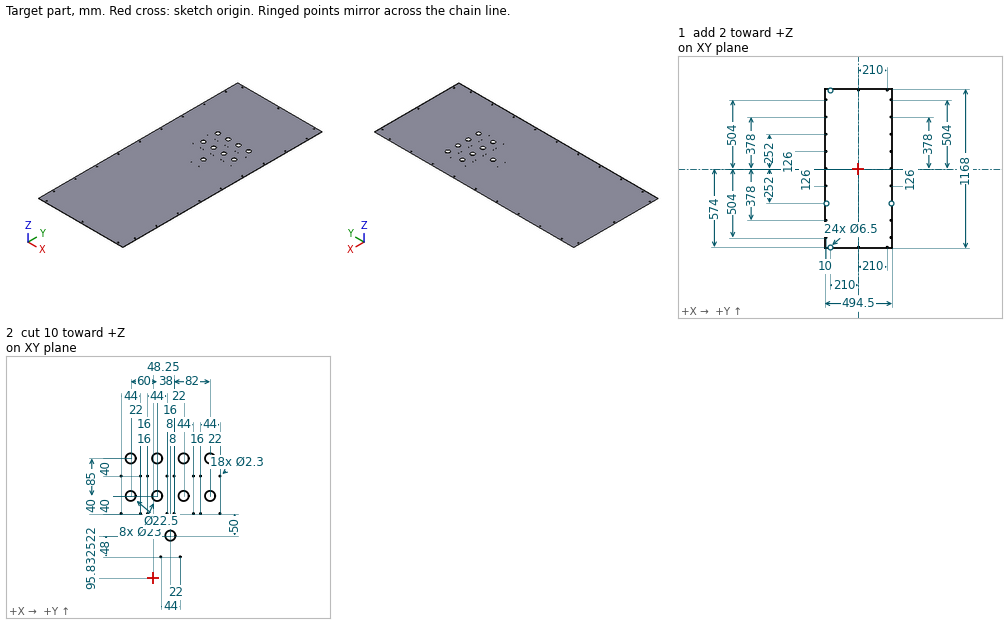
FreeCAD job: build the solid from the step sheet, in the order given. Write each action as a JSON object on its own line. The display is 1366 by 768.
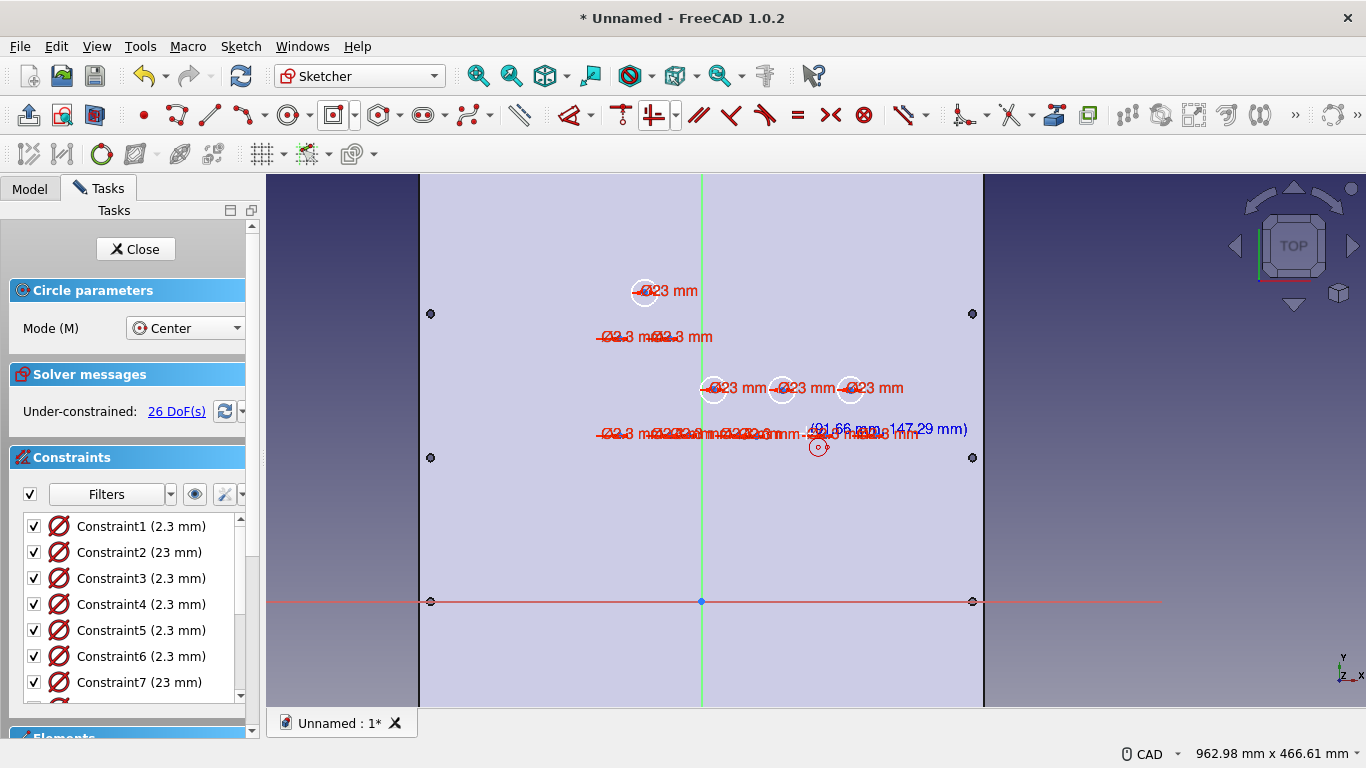
{"action": "left_click", "coordinate": [807, 435]}
{"action": "mouse_move", "coordinate": [808, 434]}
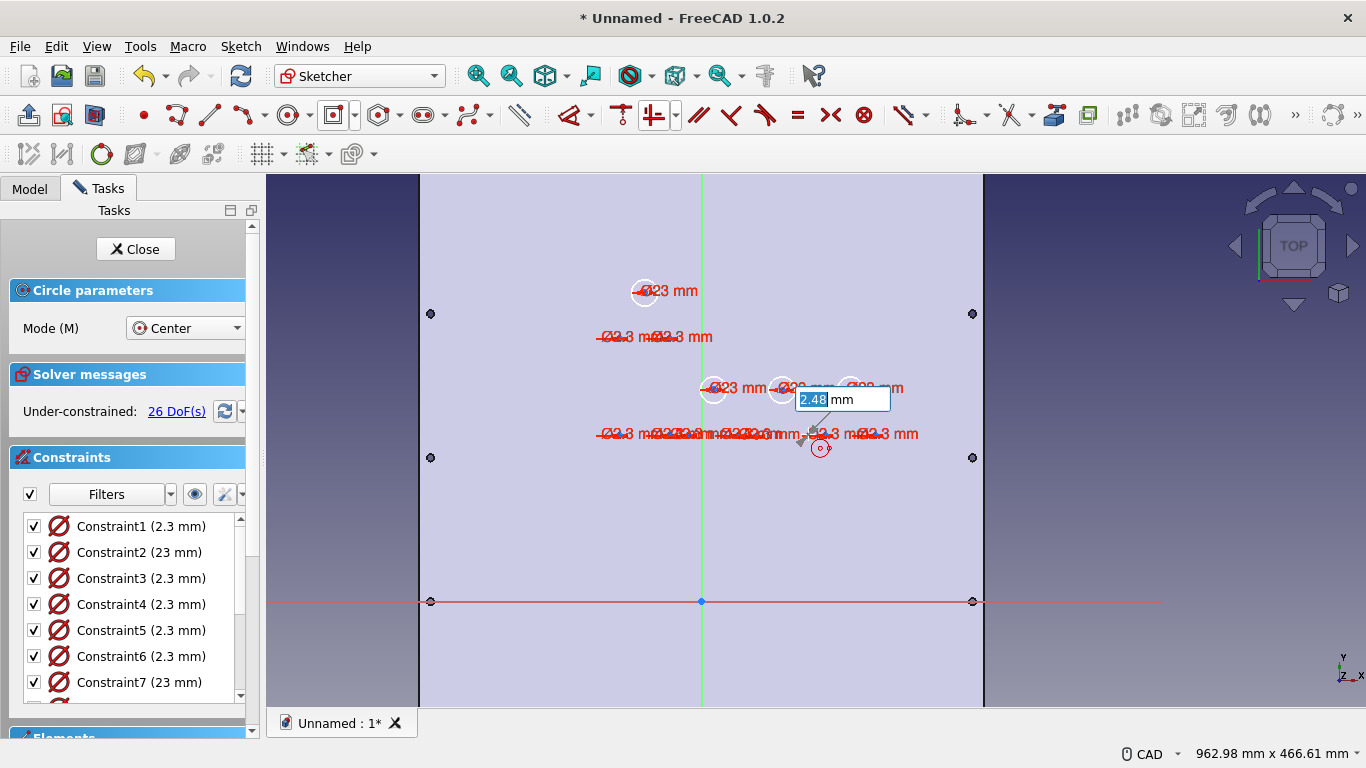
{"action": "type", "text": "2.3"}
{"action": "key", "text": "Return"}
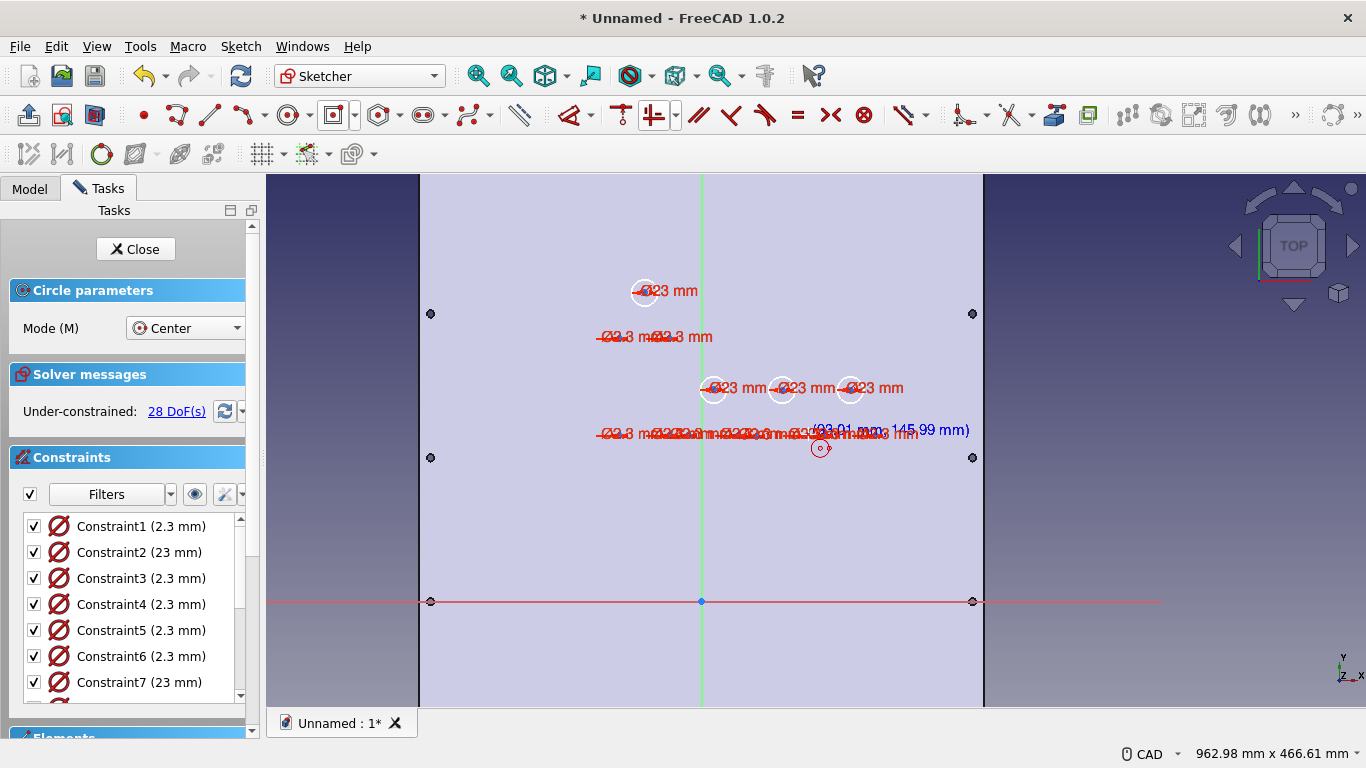
{"action": "scroll", "coordinate": [876, 338], "scroll_direction": "up", "scroll_amount": 15}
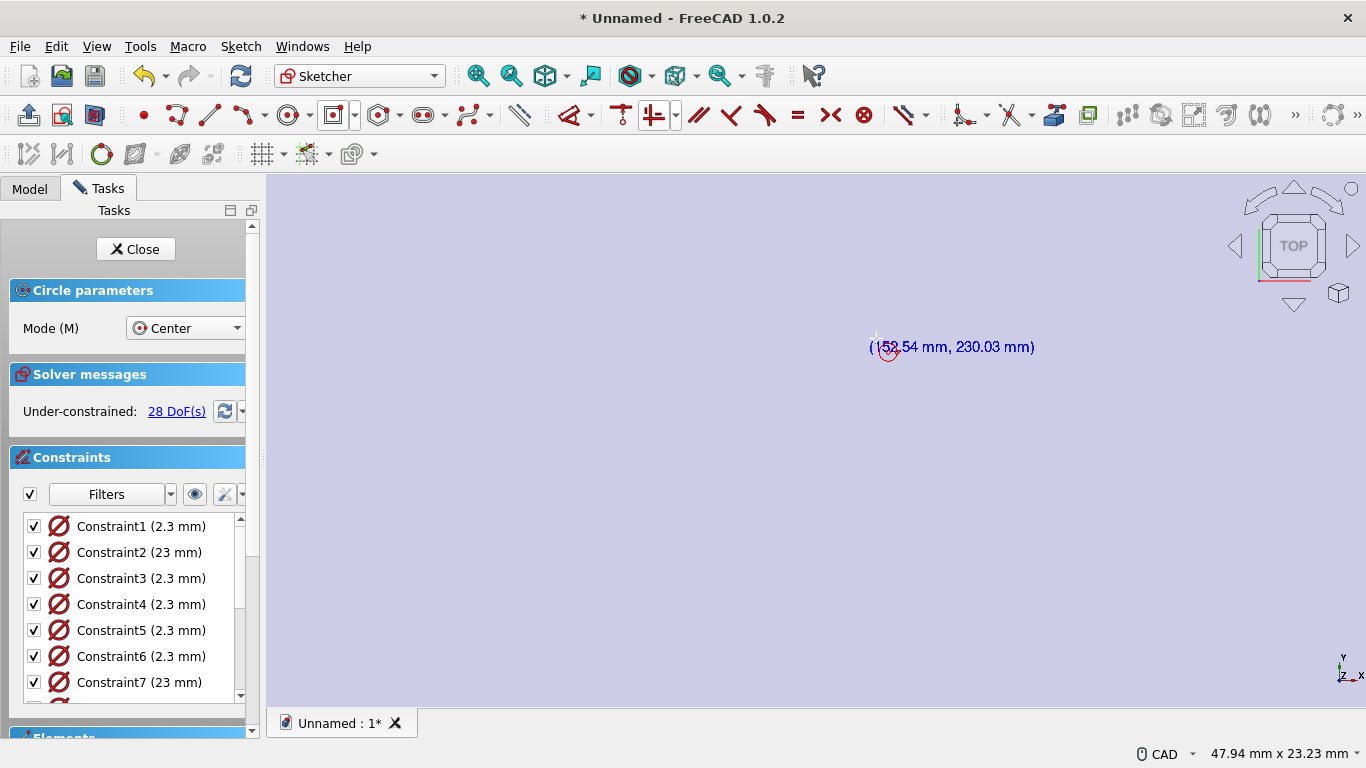
{"action": "scroll", "coordinate": [876, 338], "scroll_direction": "down", "scroll_amount": 15}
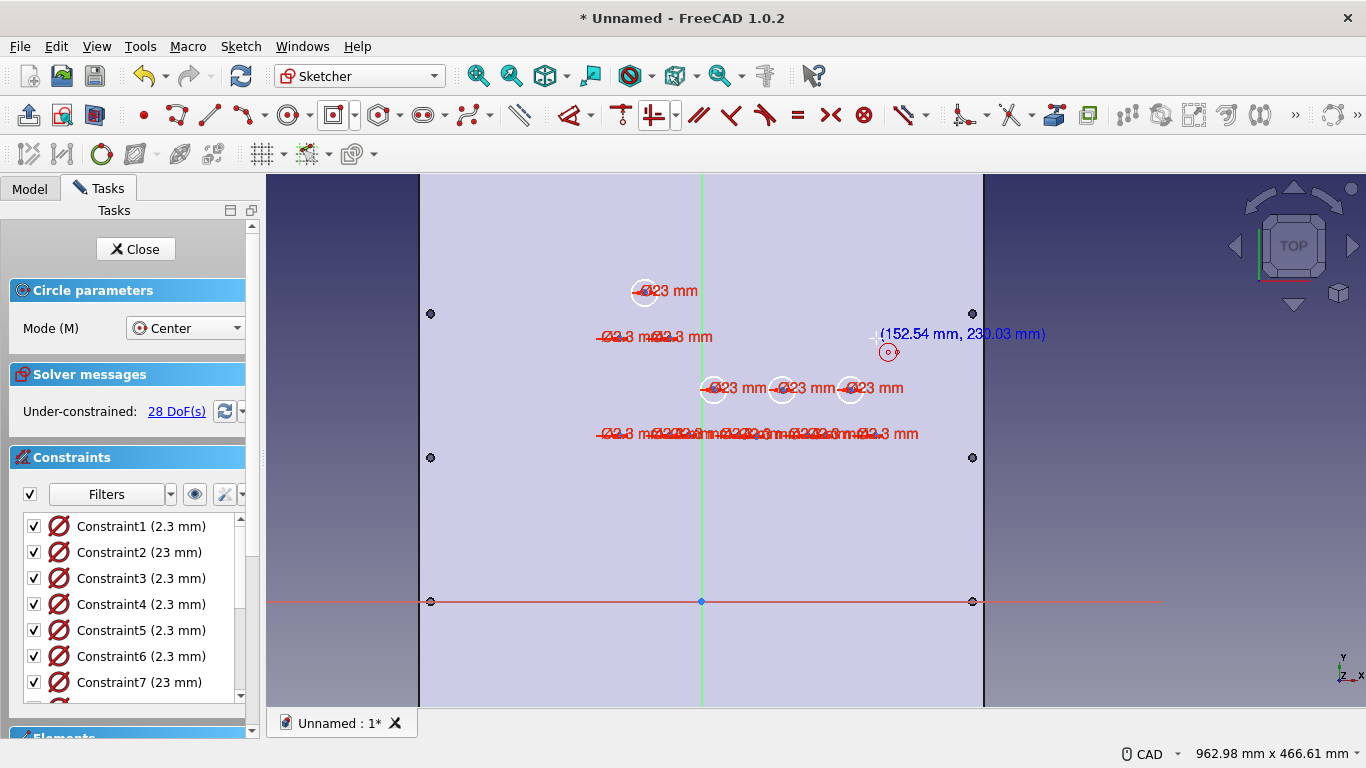
{"action": "left_click", "coordinate": [876, 338]}
{"action": "mouse_move", "coordinate": [877, 337]}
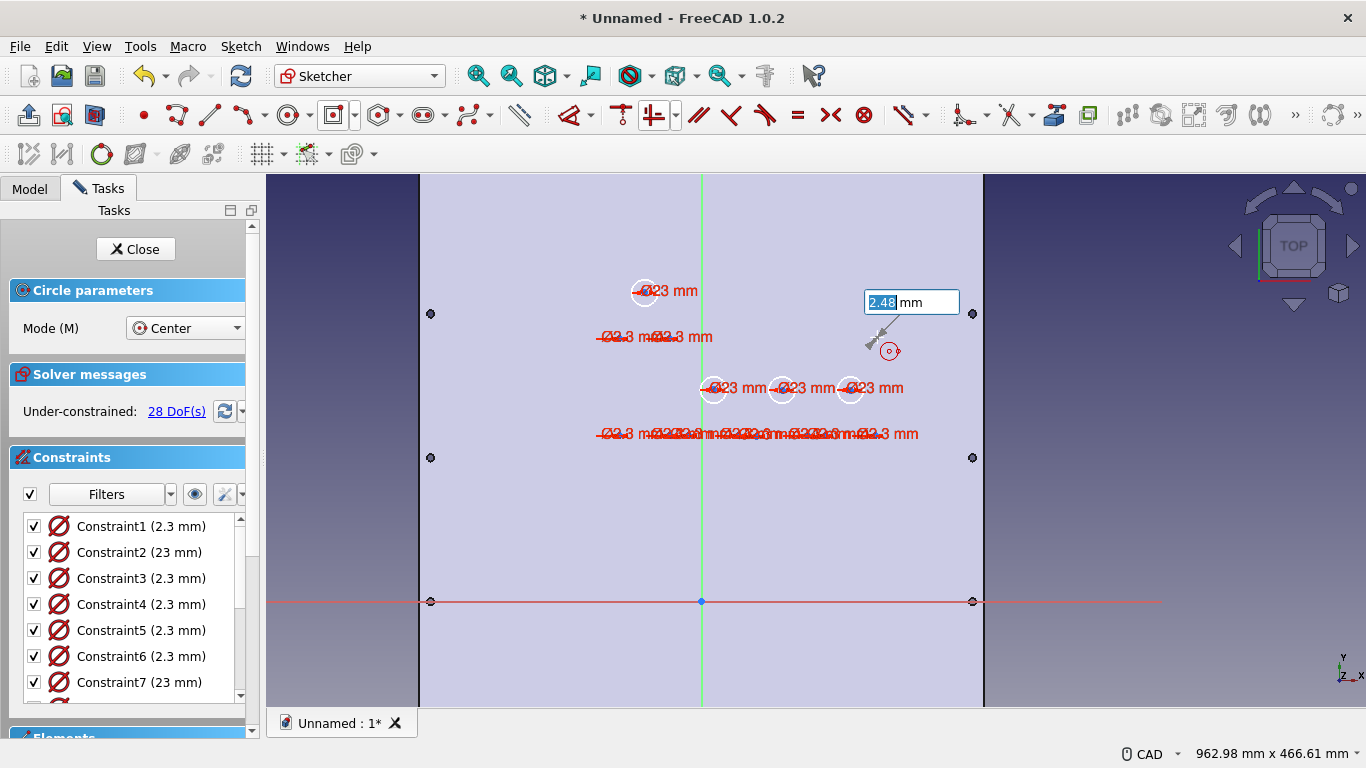
{"action": "type", "text": "2.3"}
{"action": "key", "text": "Return"}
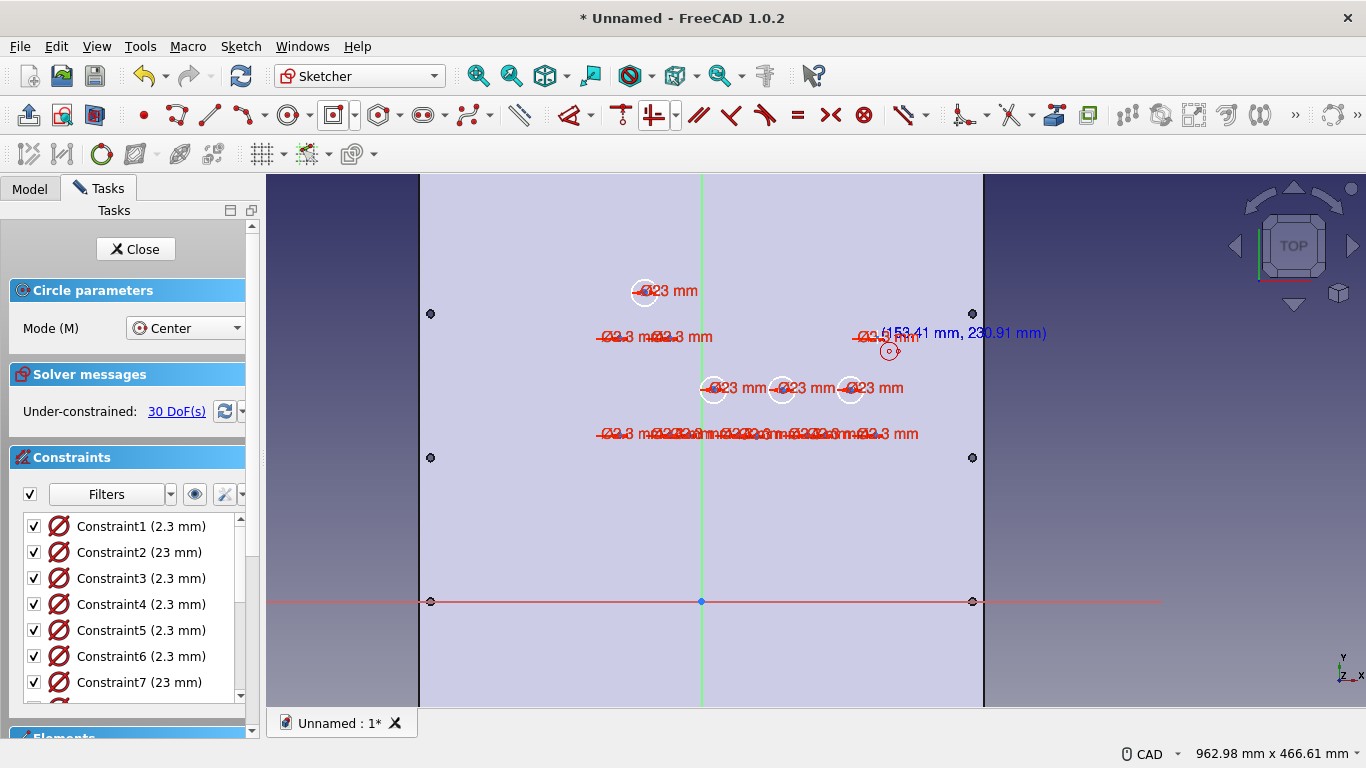
{"action": "scroll", "coordinate": [825, 338], "scroll_direction": "up", "scroll_amount": 15}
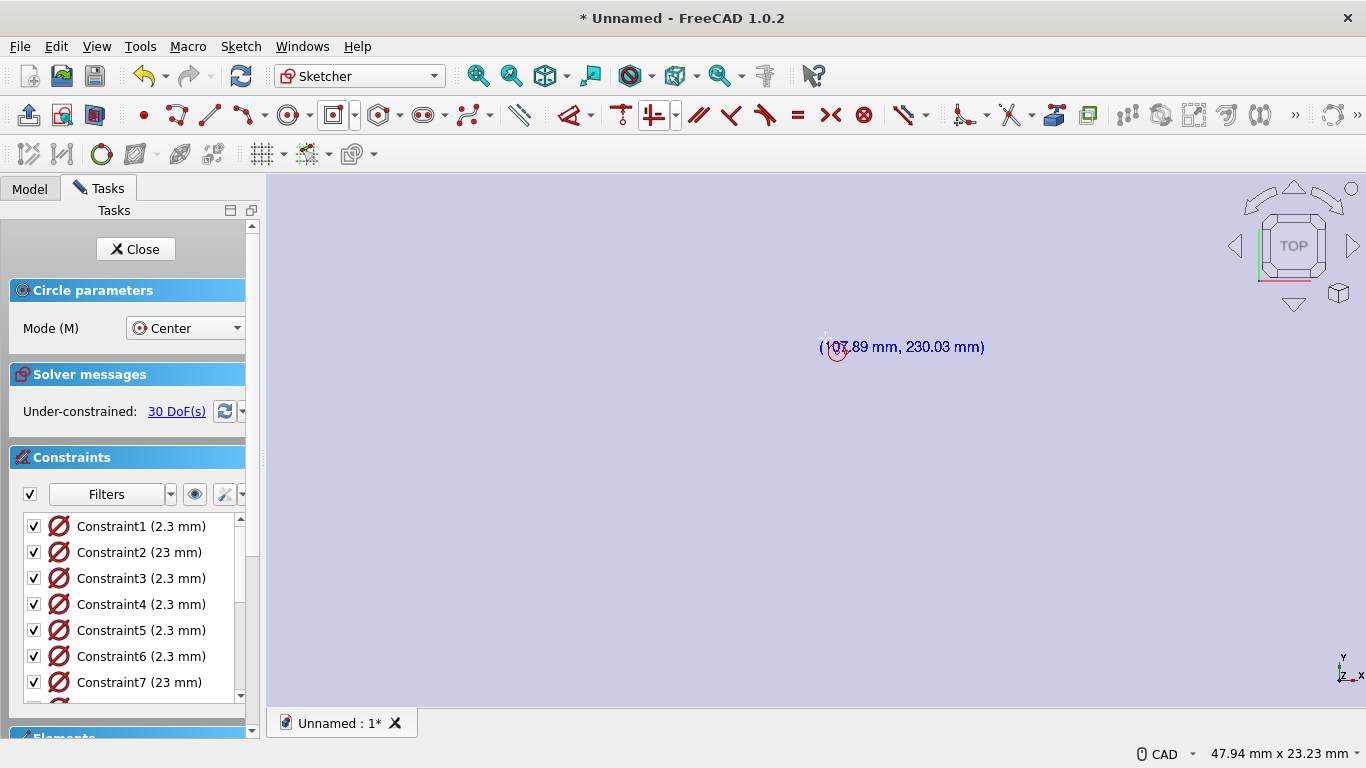
{"action": "scroll", "coordinate": [825, 338], "scroll_direction": "down", "scroll_amount": 15}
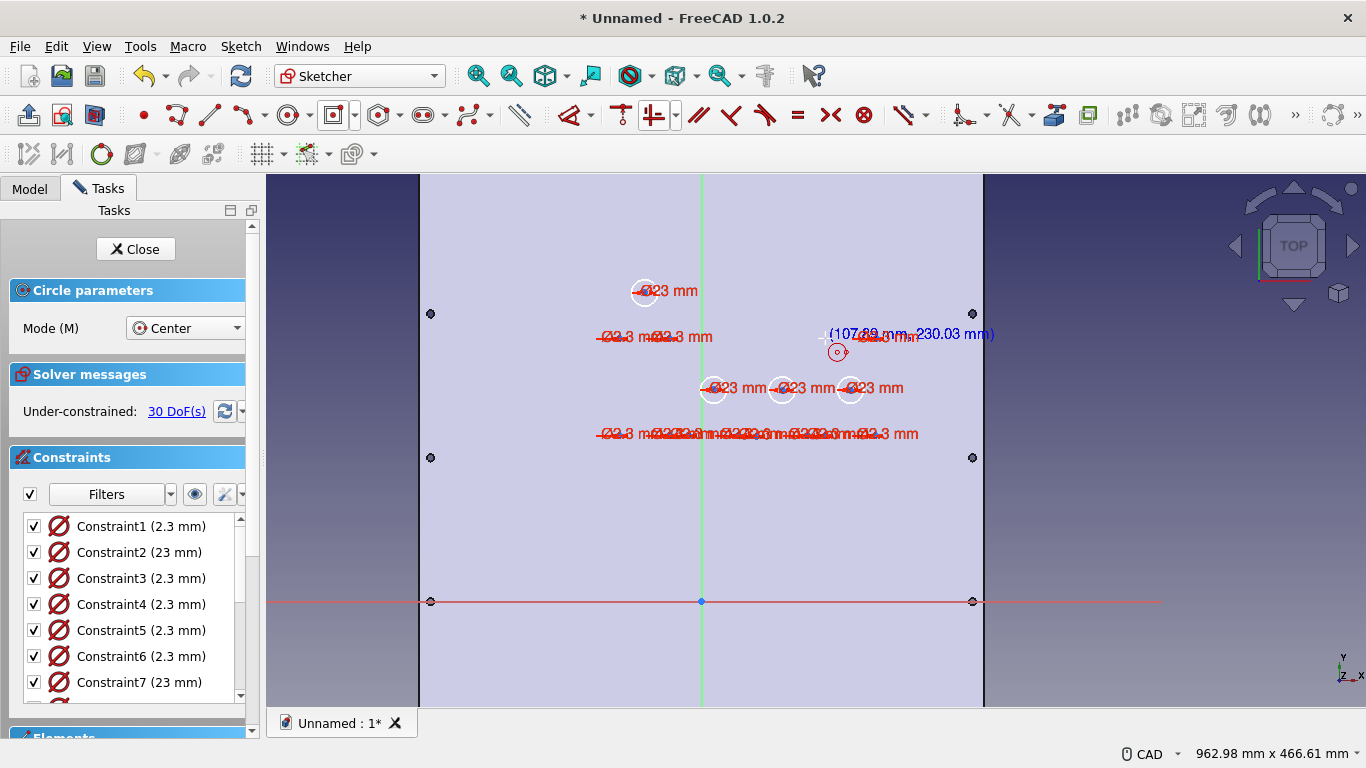
{"action": "left_click", "coordinate": [825, 338]}
{"action": "mouse_move", "coordinate": [826, 337]}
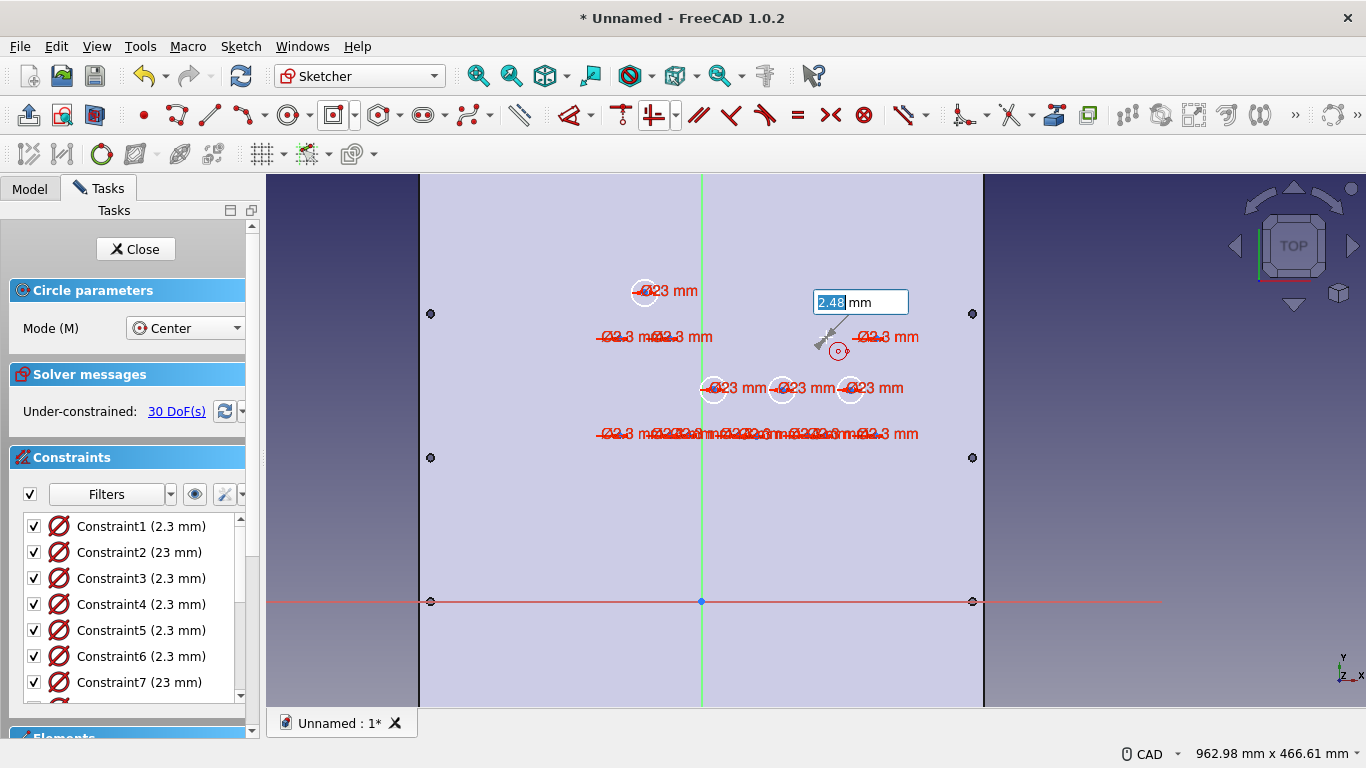
{"action": "type", "text": "2.3"}
{"action": "key", "text": "Return"}